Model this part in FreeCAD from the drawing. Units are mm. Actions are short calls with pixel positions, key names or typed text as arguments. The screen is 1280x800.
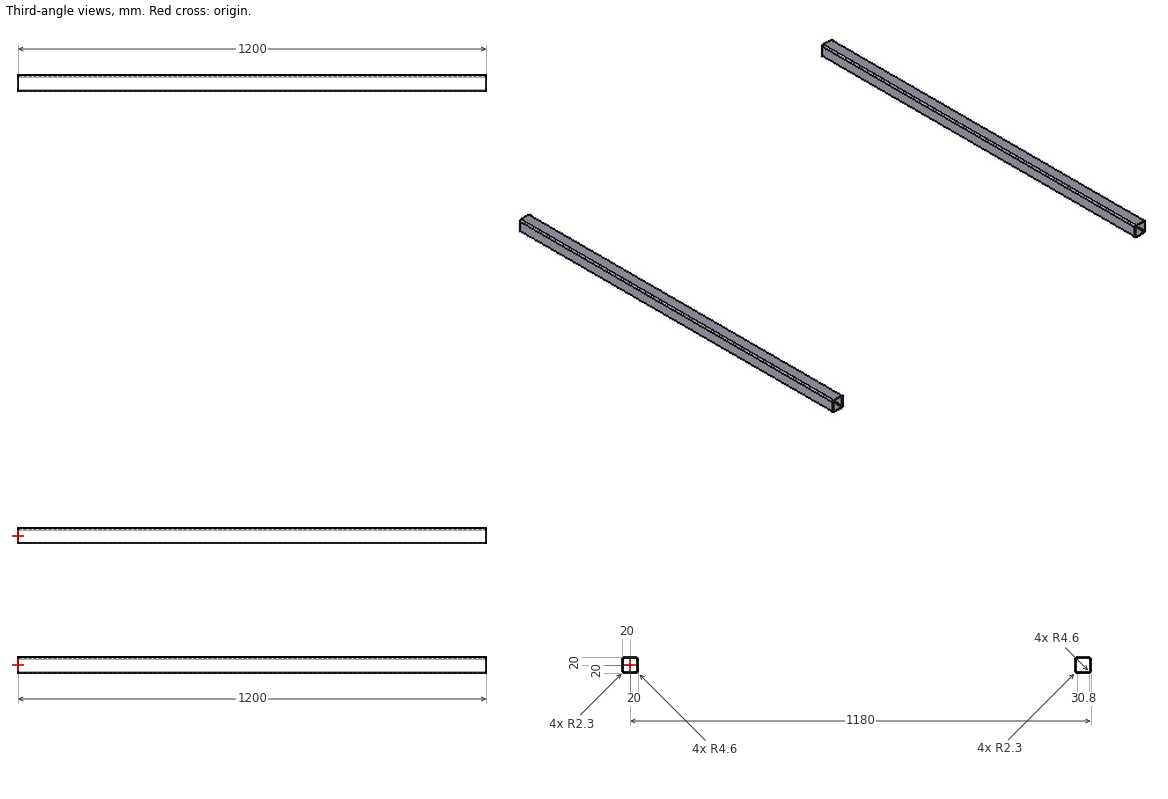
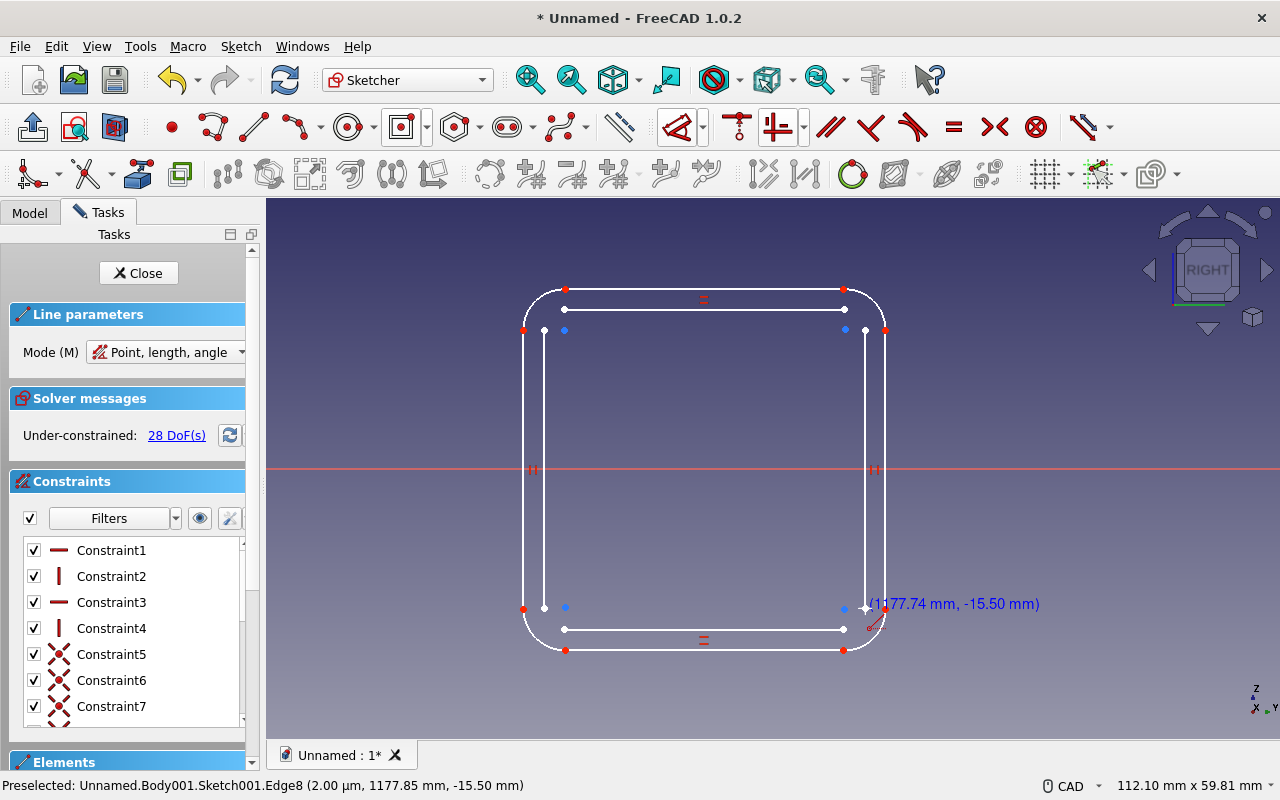
key(g)
key(3)
key(a)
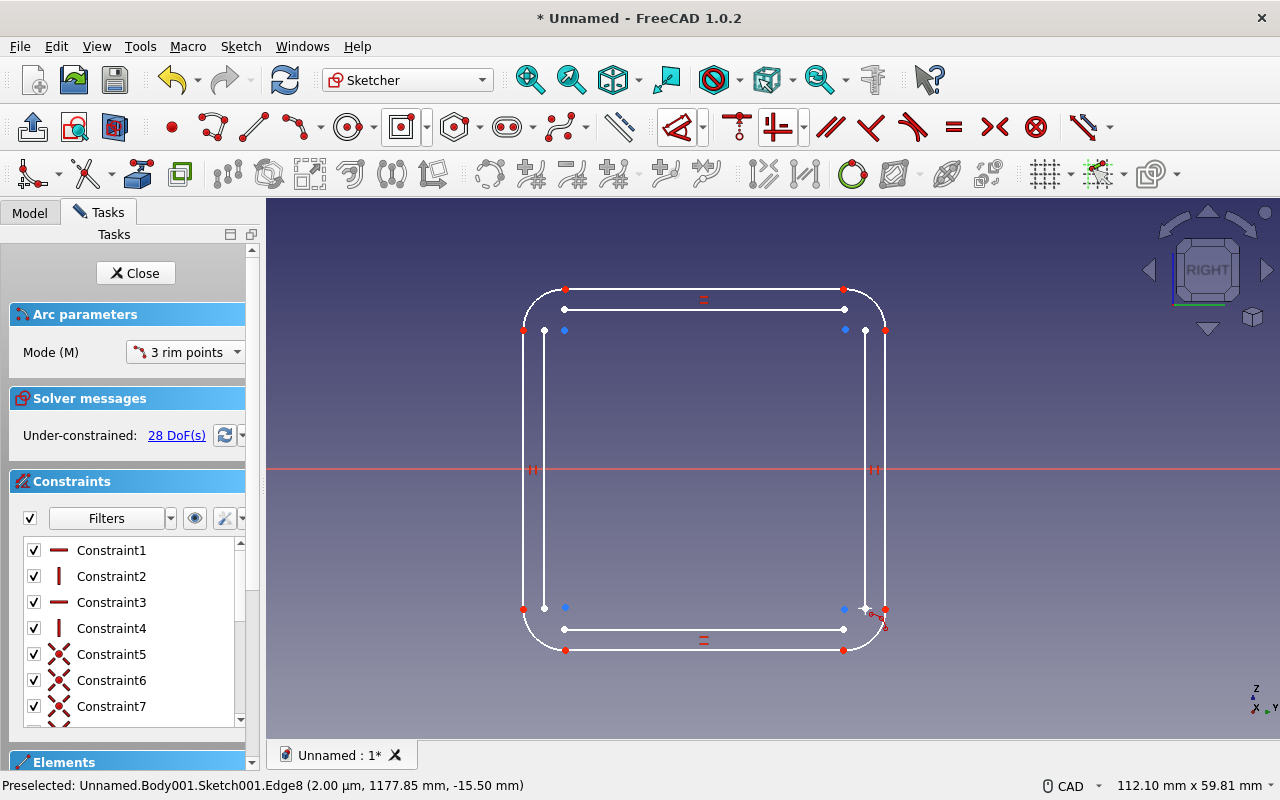
click(565, 630)
click(544, 609)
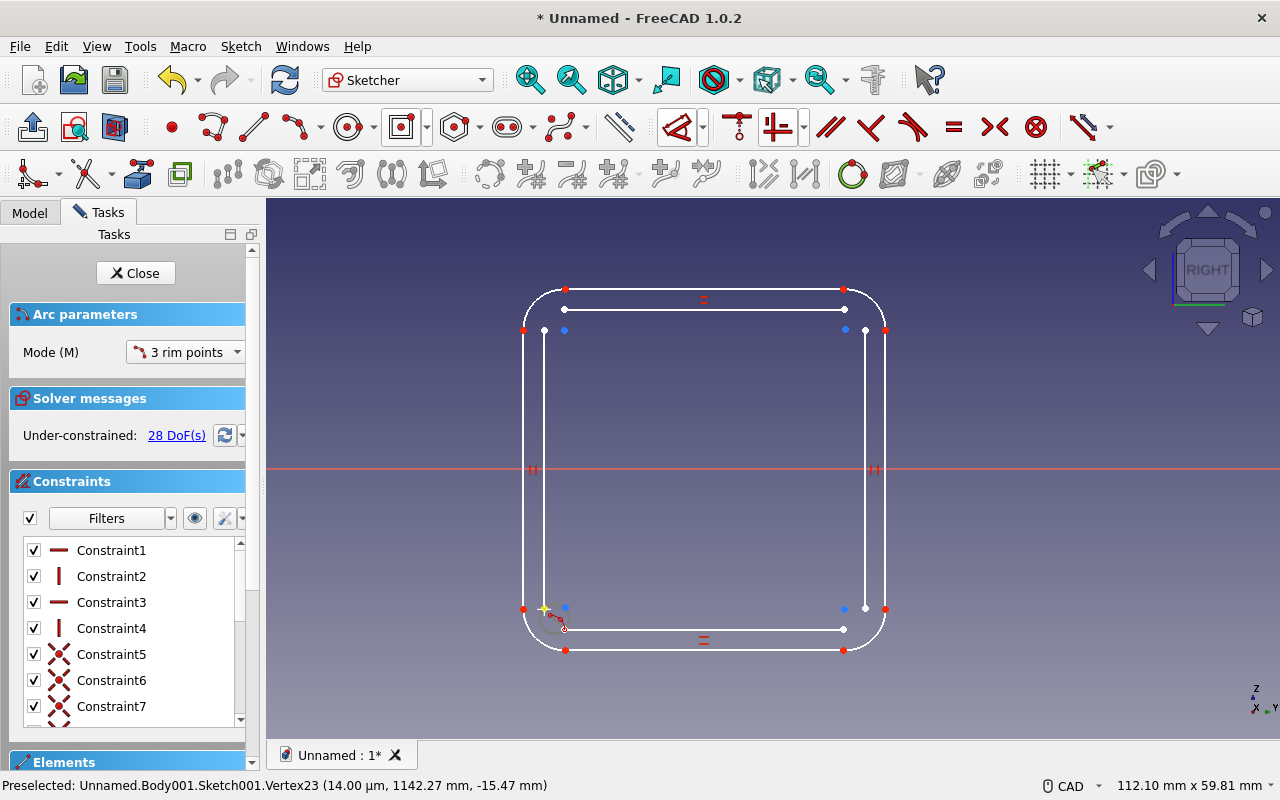
scroll(551, 623, up, 5)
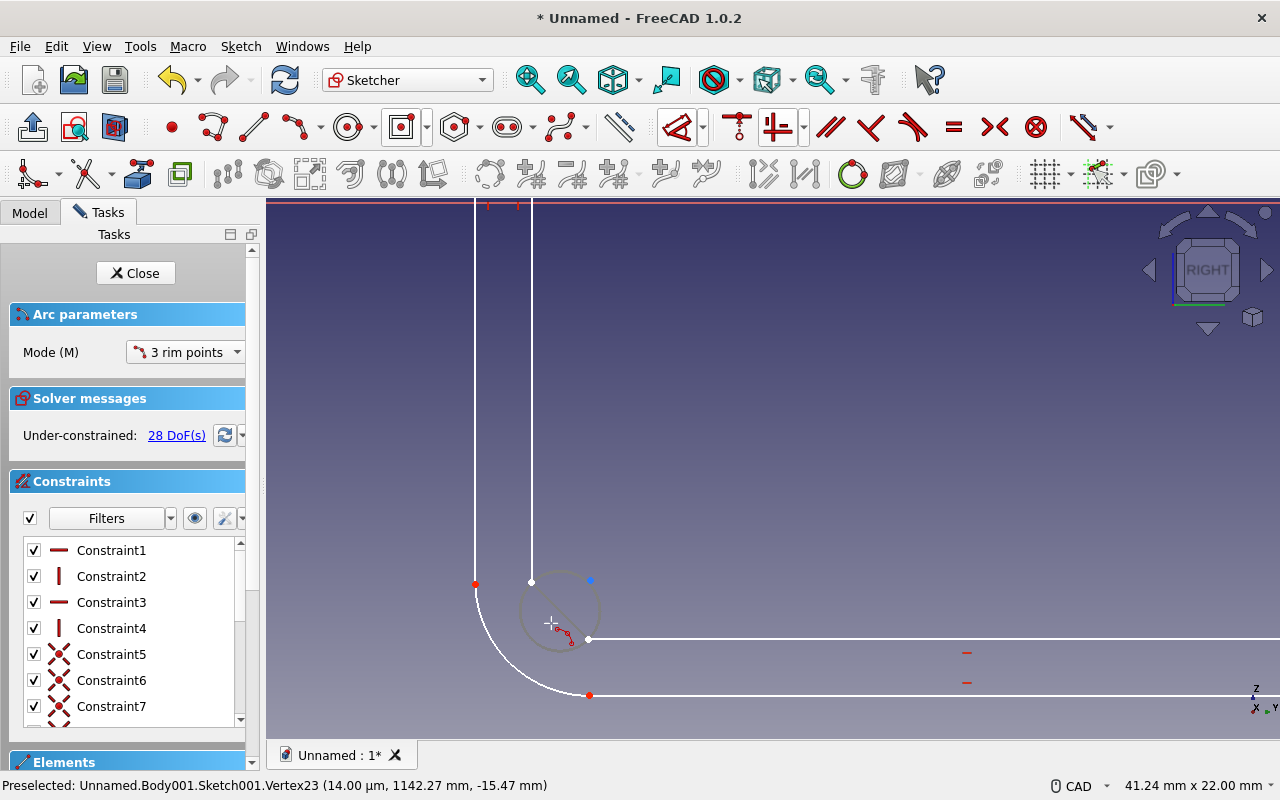
click(549, 621)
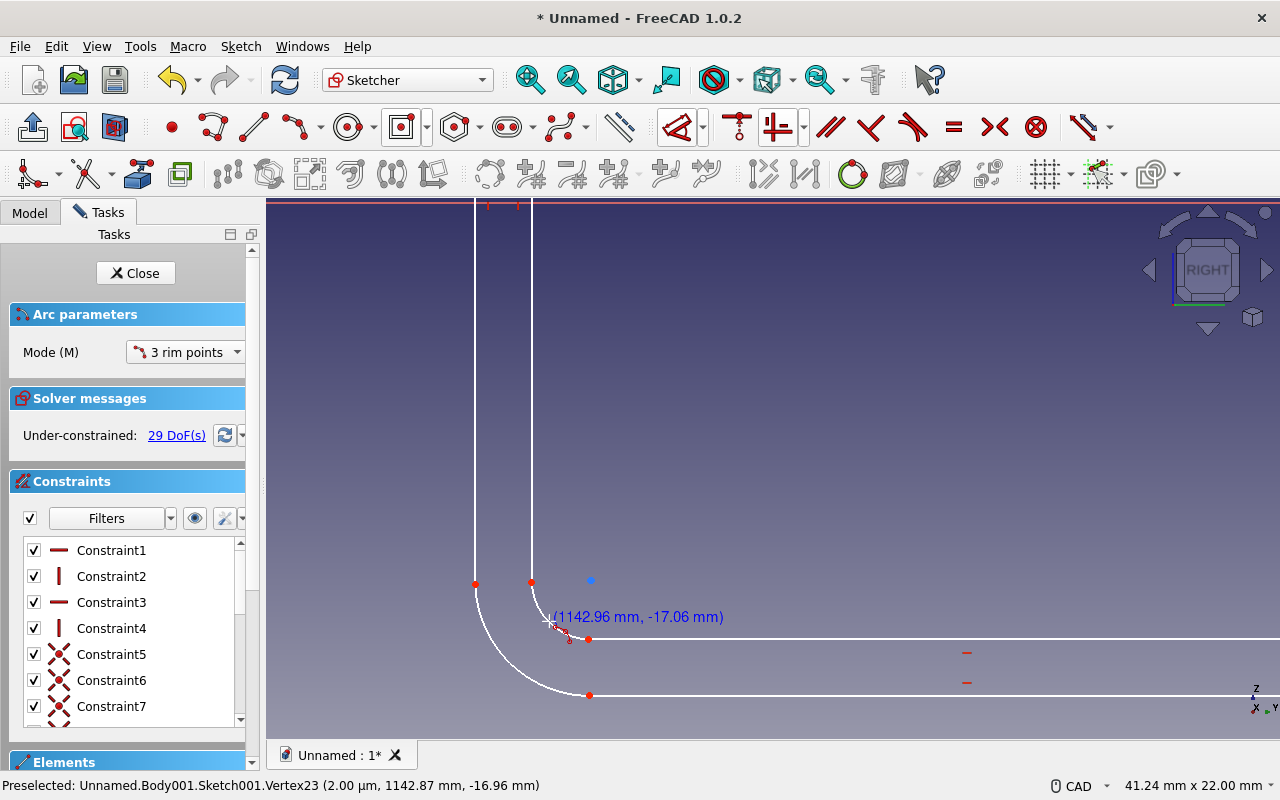
scroll(551, 623, down, 5)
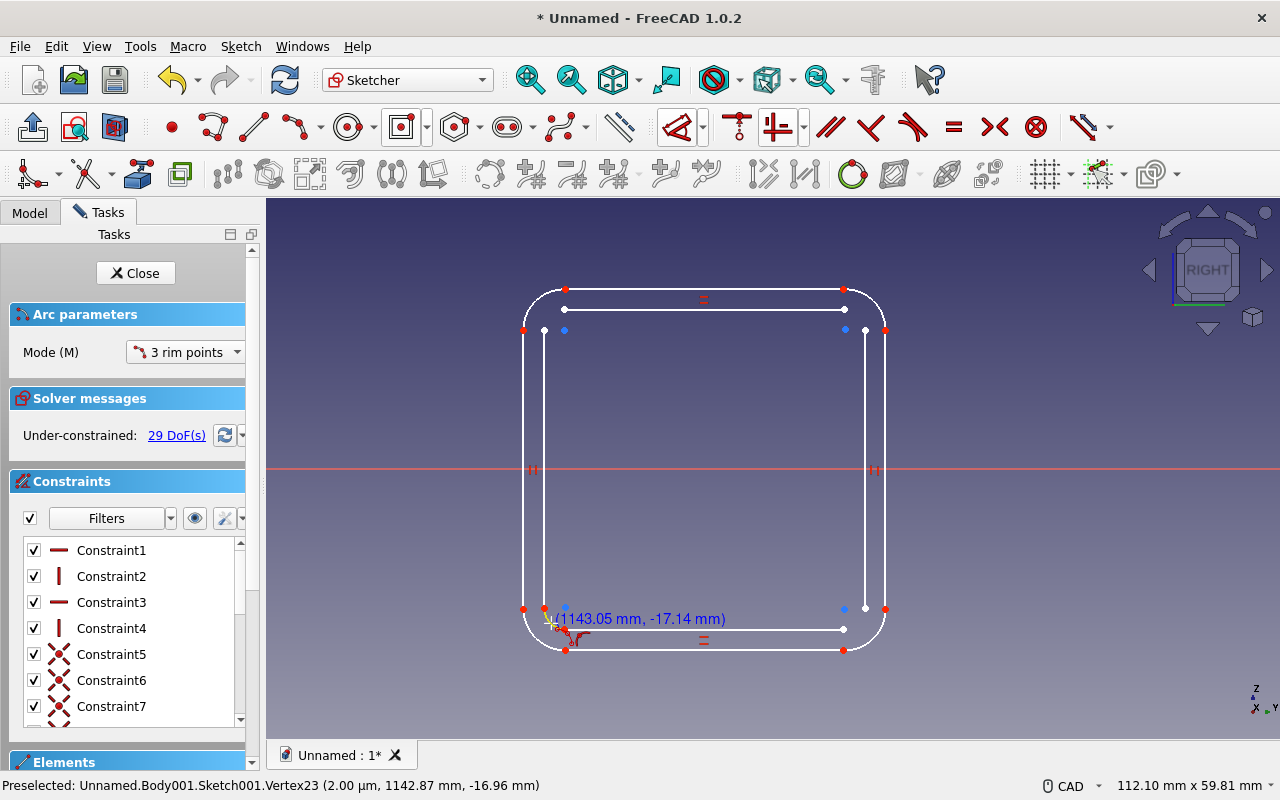
click(544, 331)
click(565, 310)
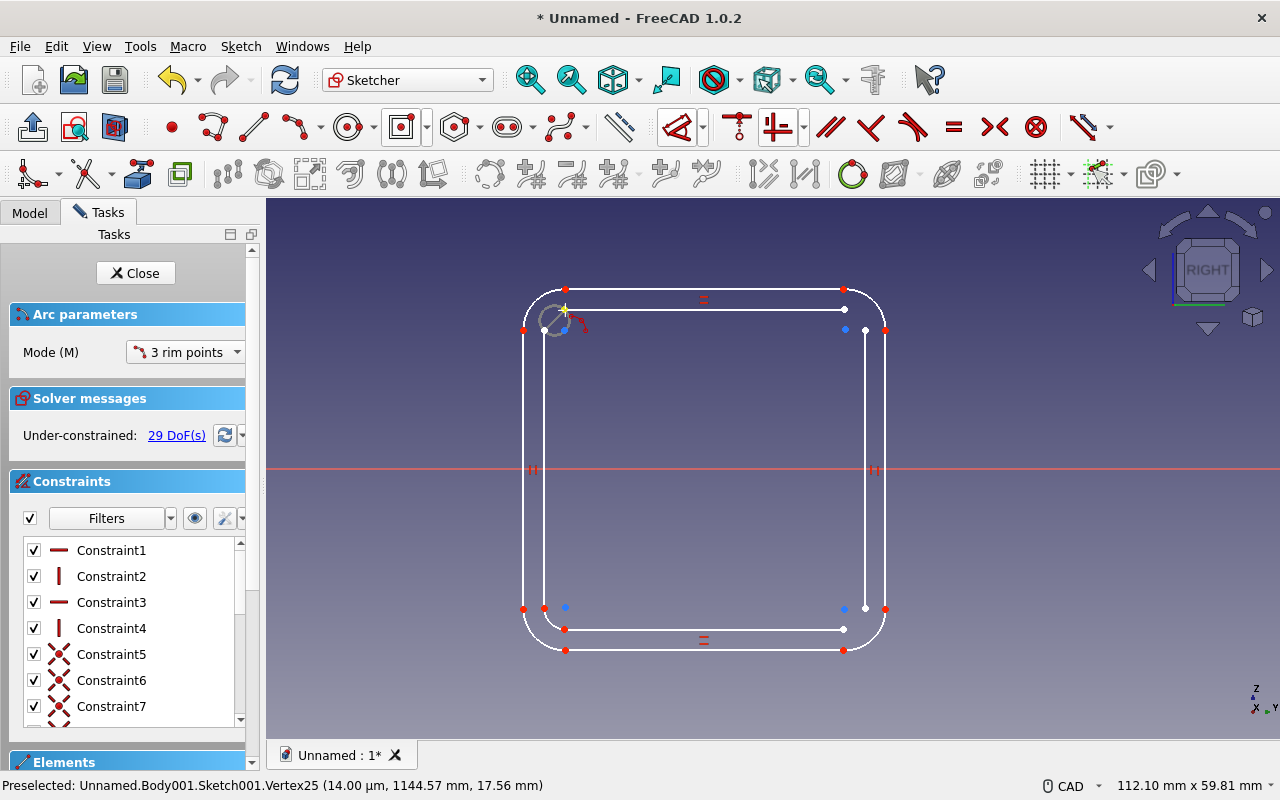
scroll(551, 315, up, 5)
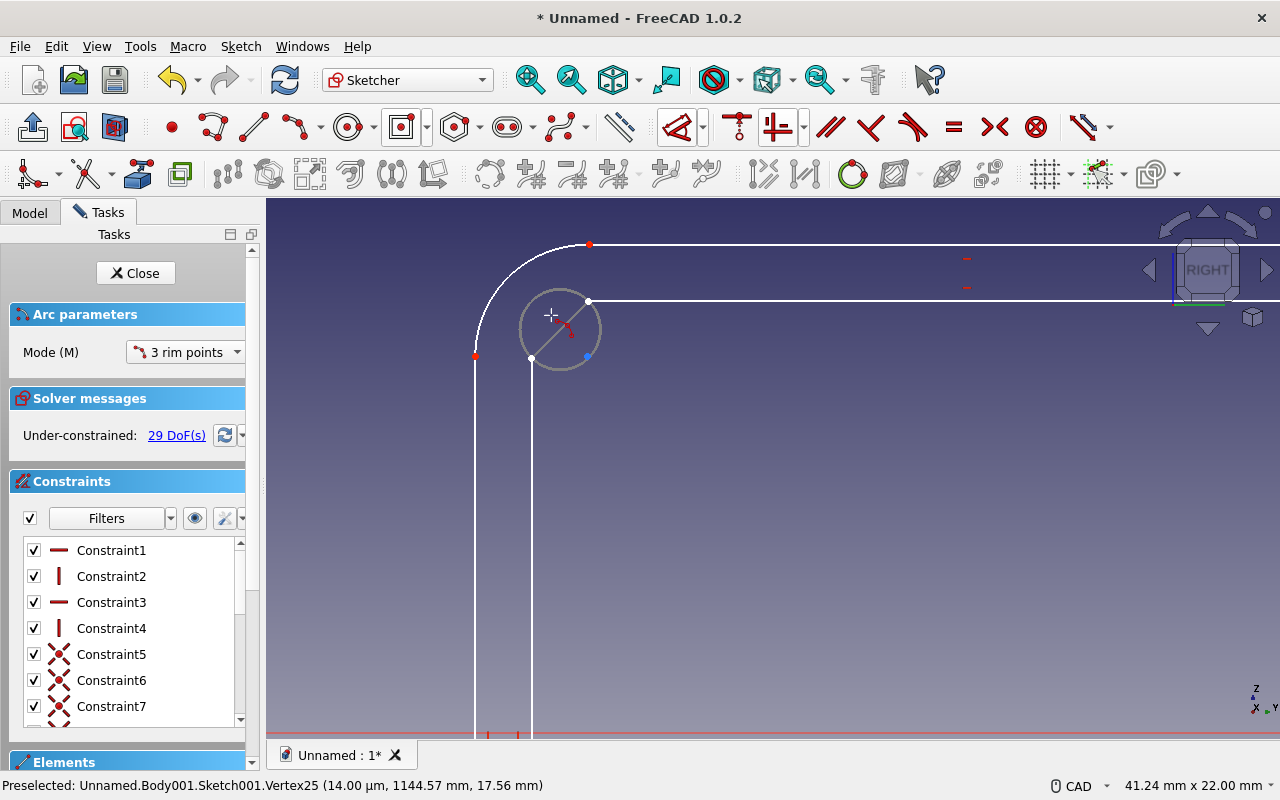
click(549, 314)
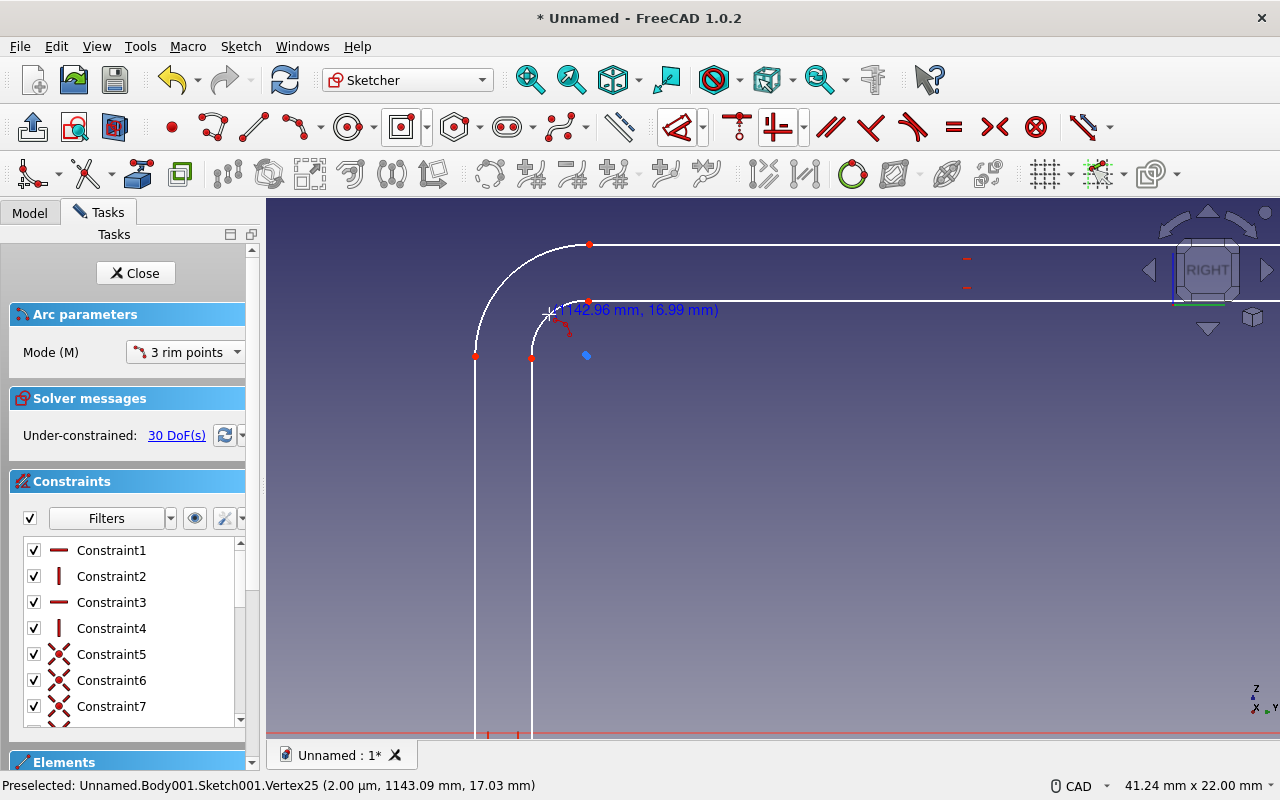
scroll(551, 315, down, 5)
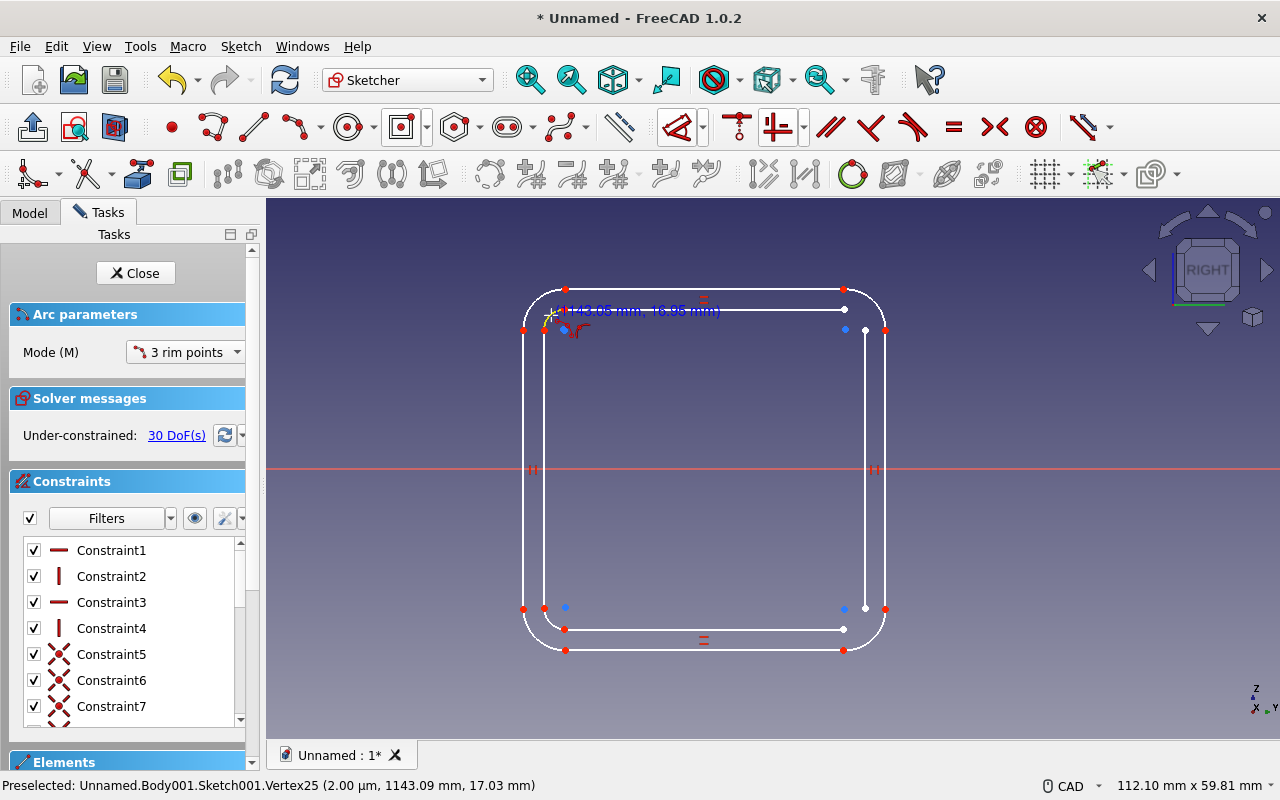
click(844, 310)
click(865, 331)